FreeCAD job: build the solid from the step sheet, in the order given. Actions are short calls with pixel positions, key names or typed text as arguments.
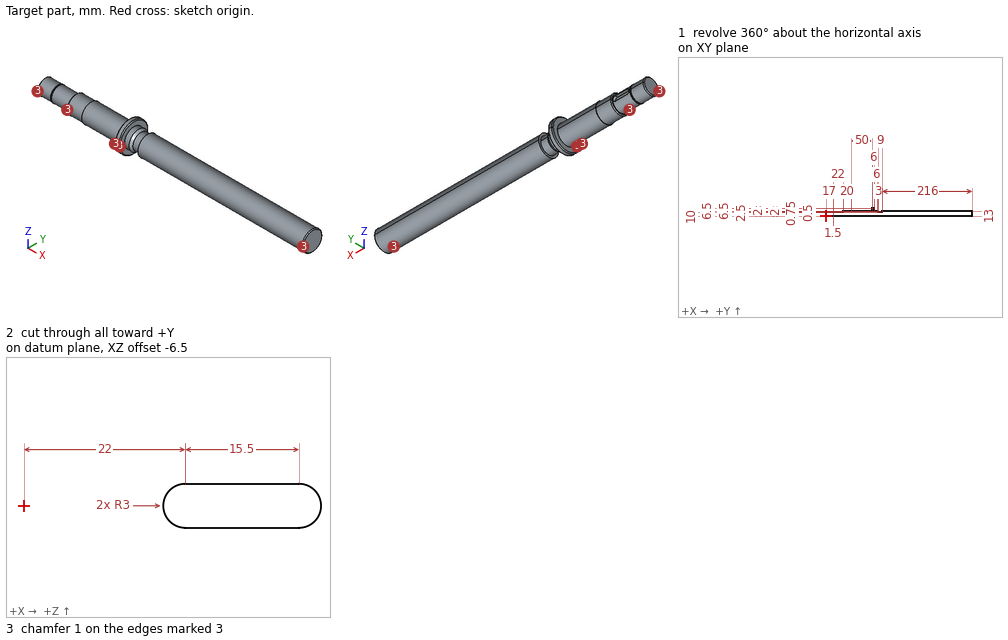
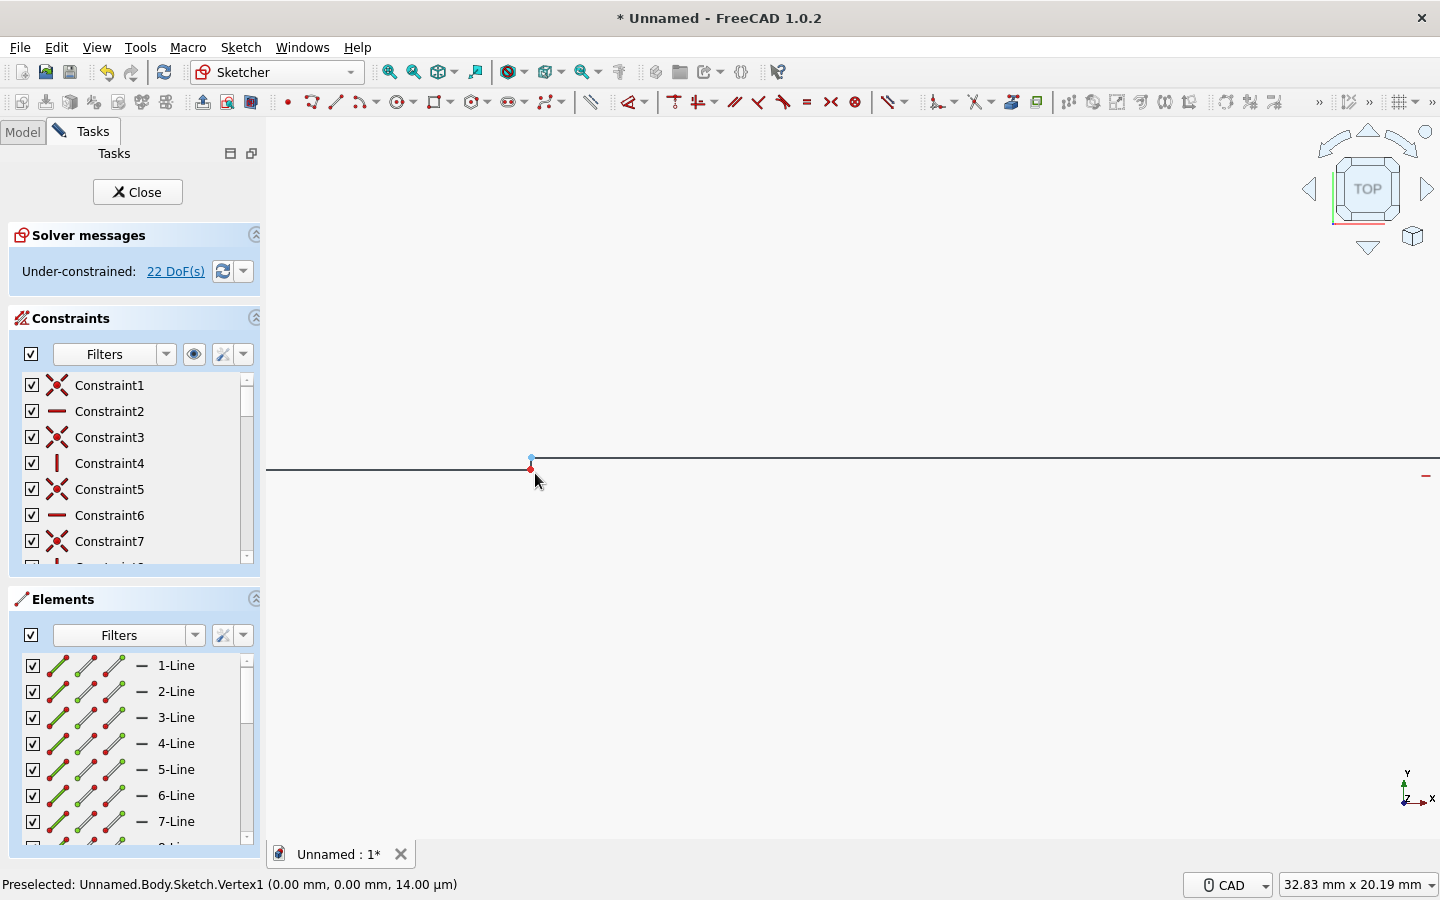
click(531, 464)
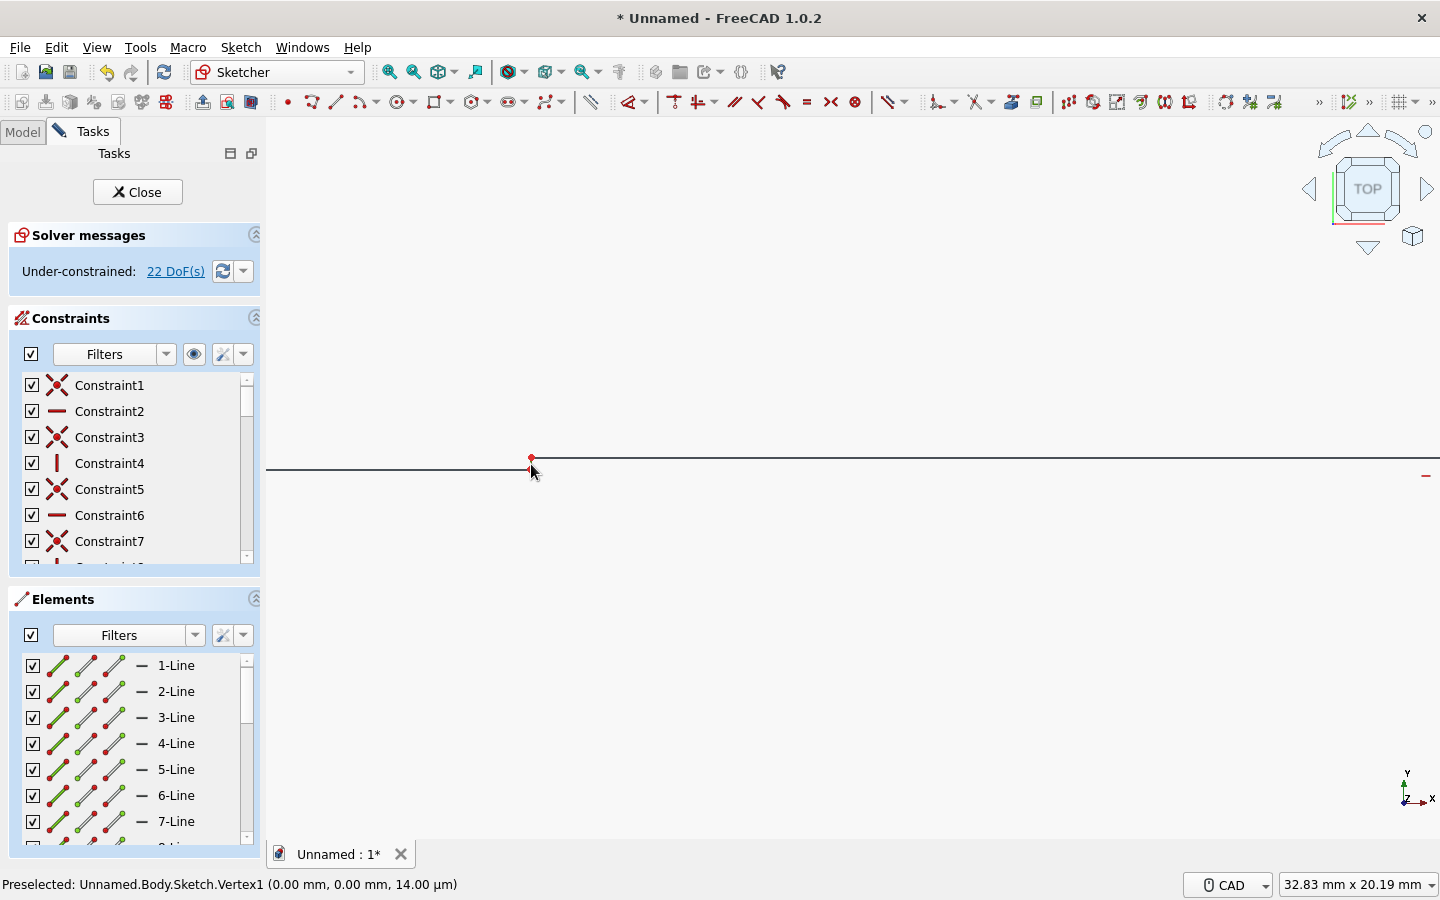
key(v)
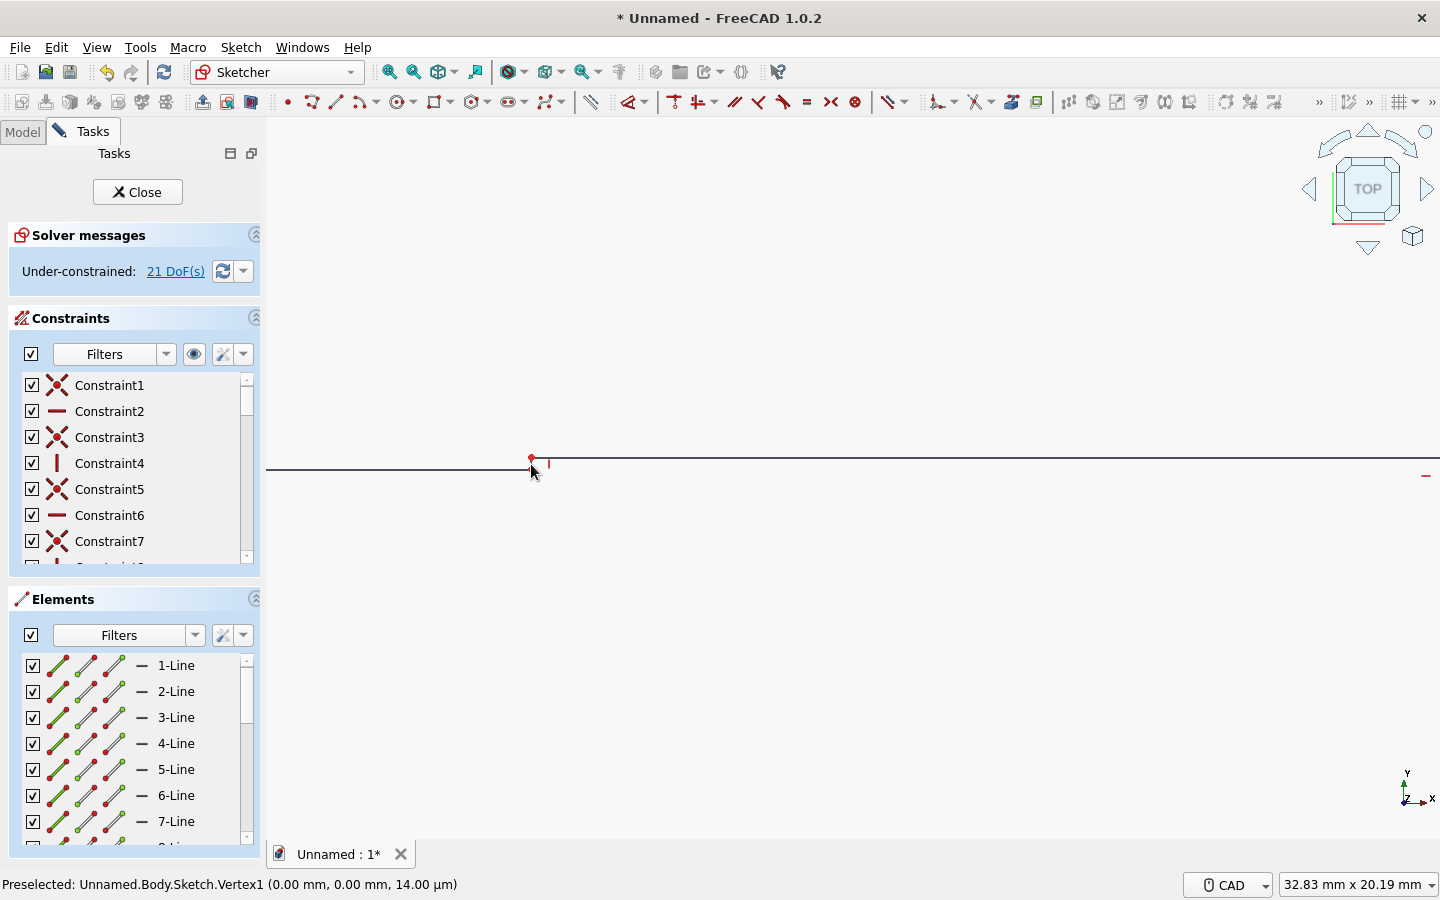
scroll(535, 473, down, 14)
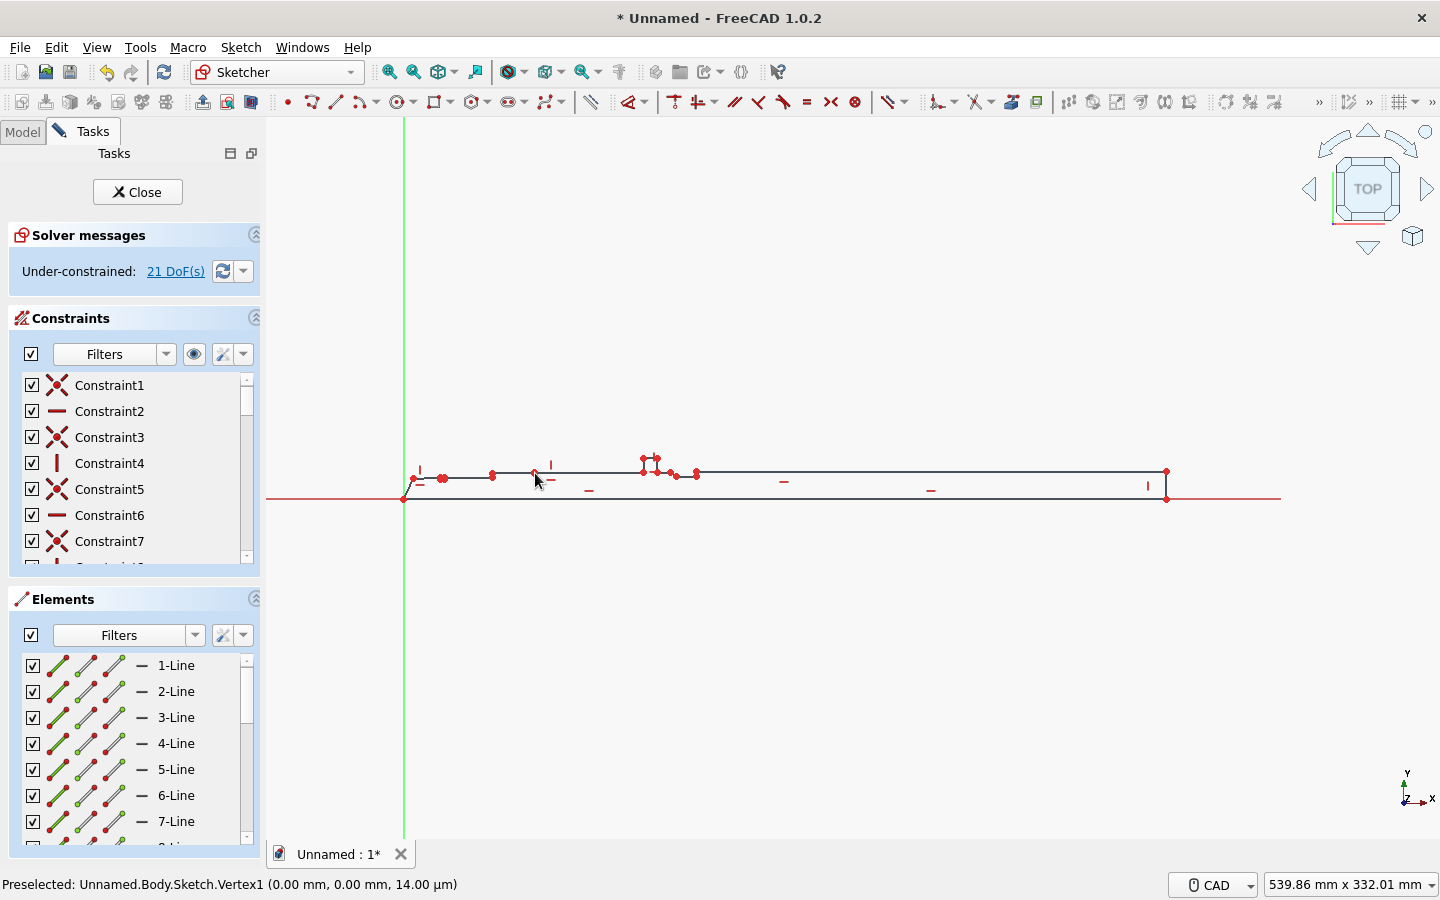
scroll(432, 478, up, 3)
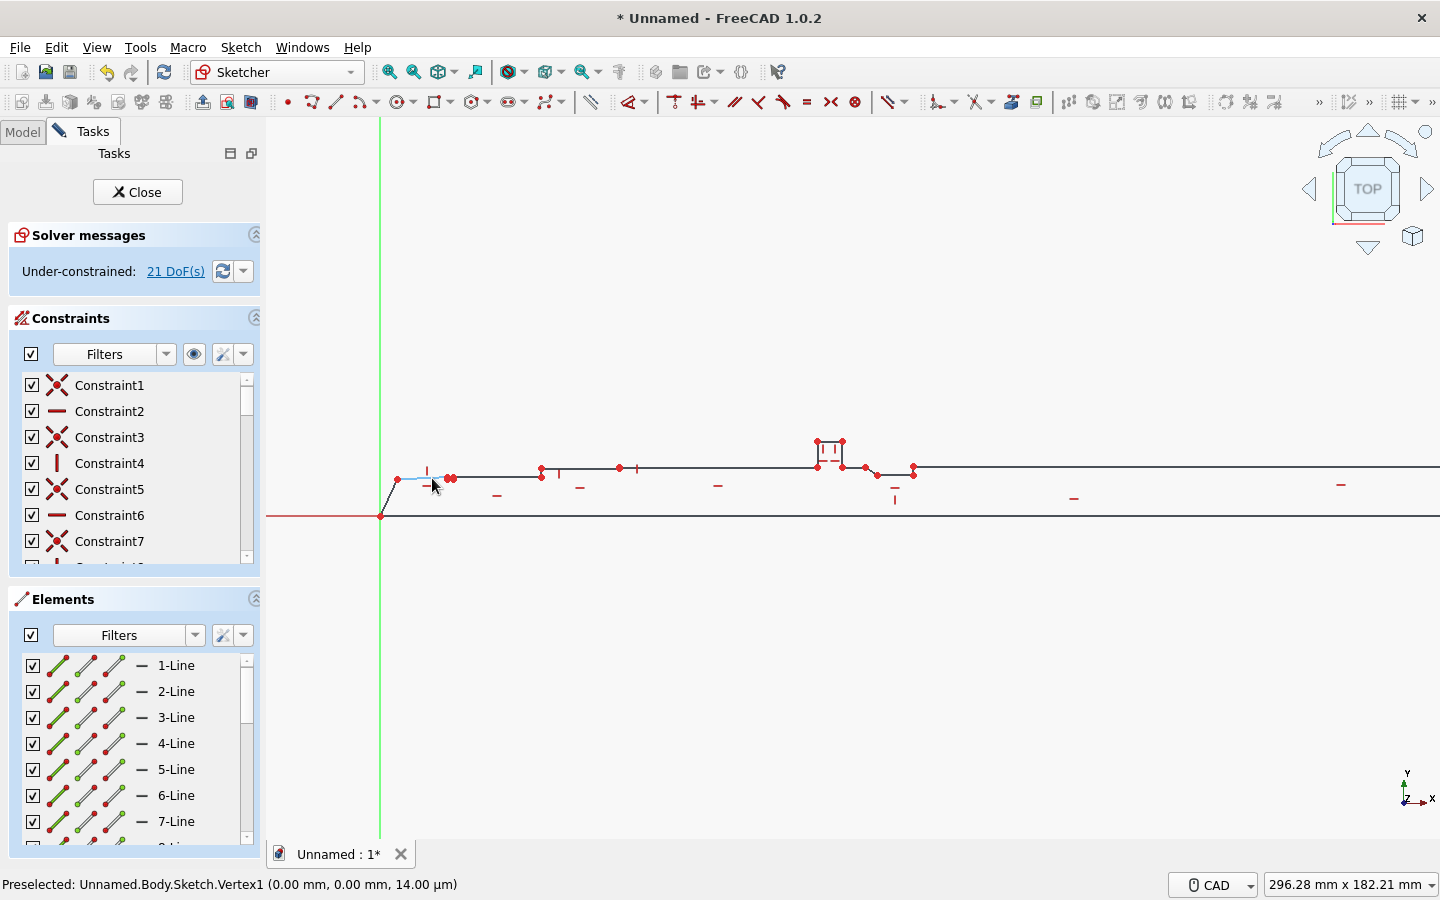
click(412, 479)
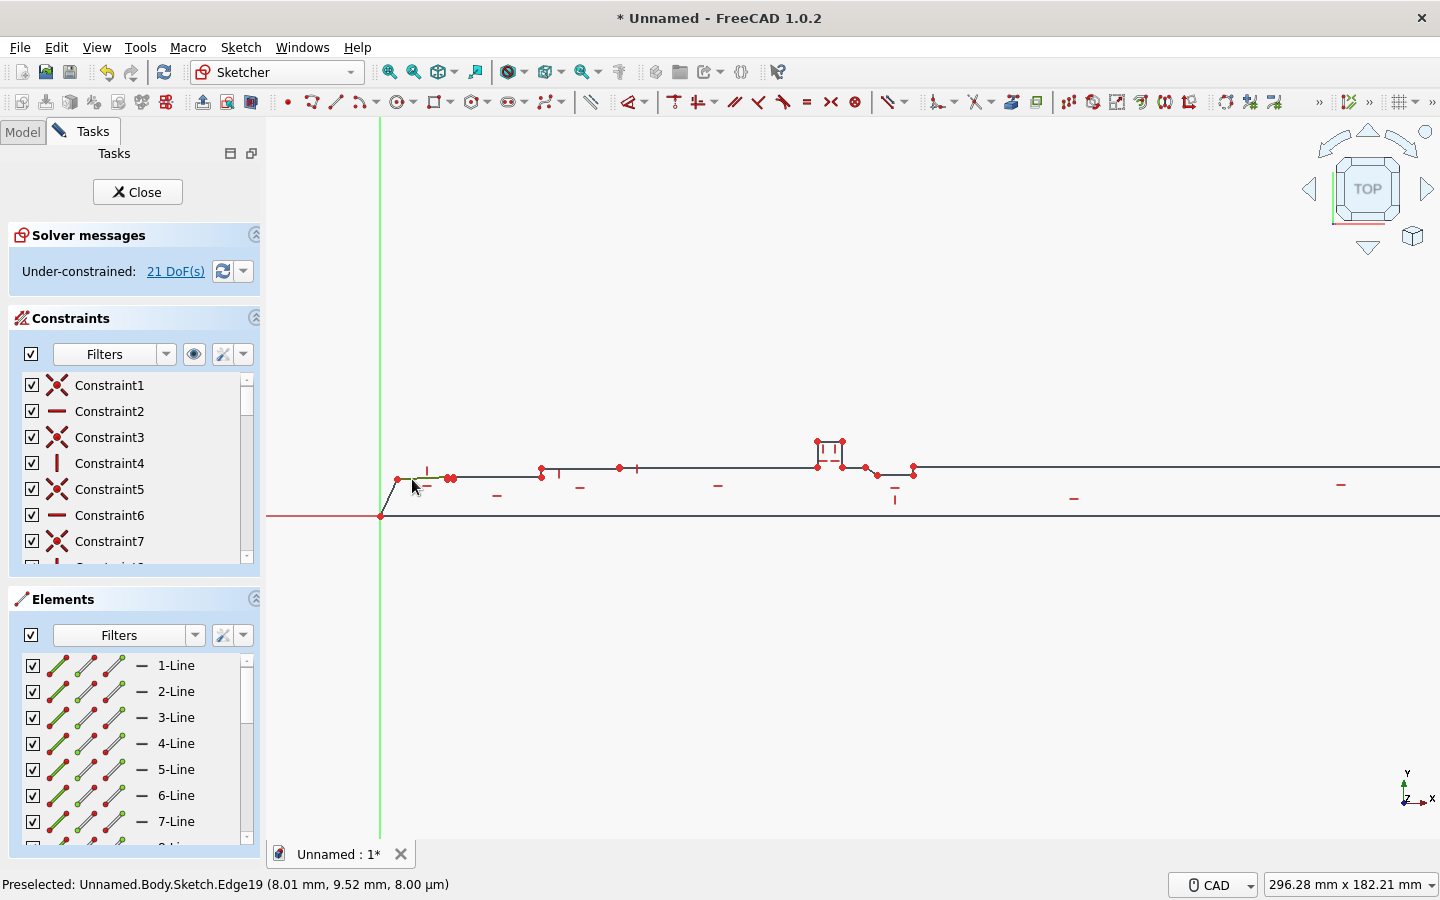
click(716, 102)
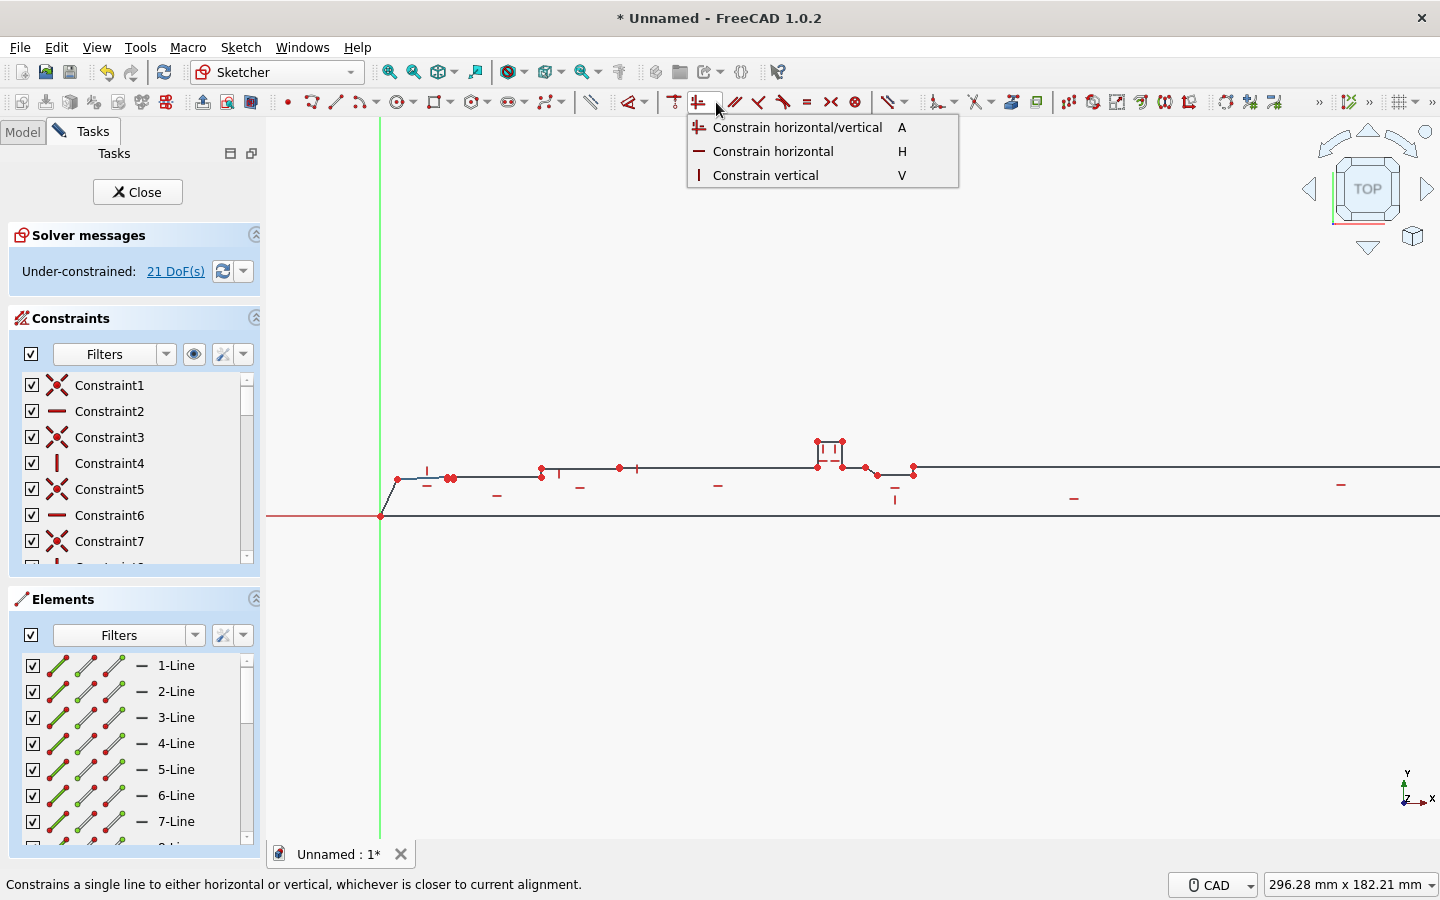
click(823, 151)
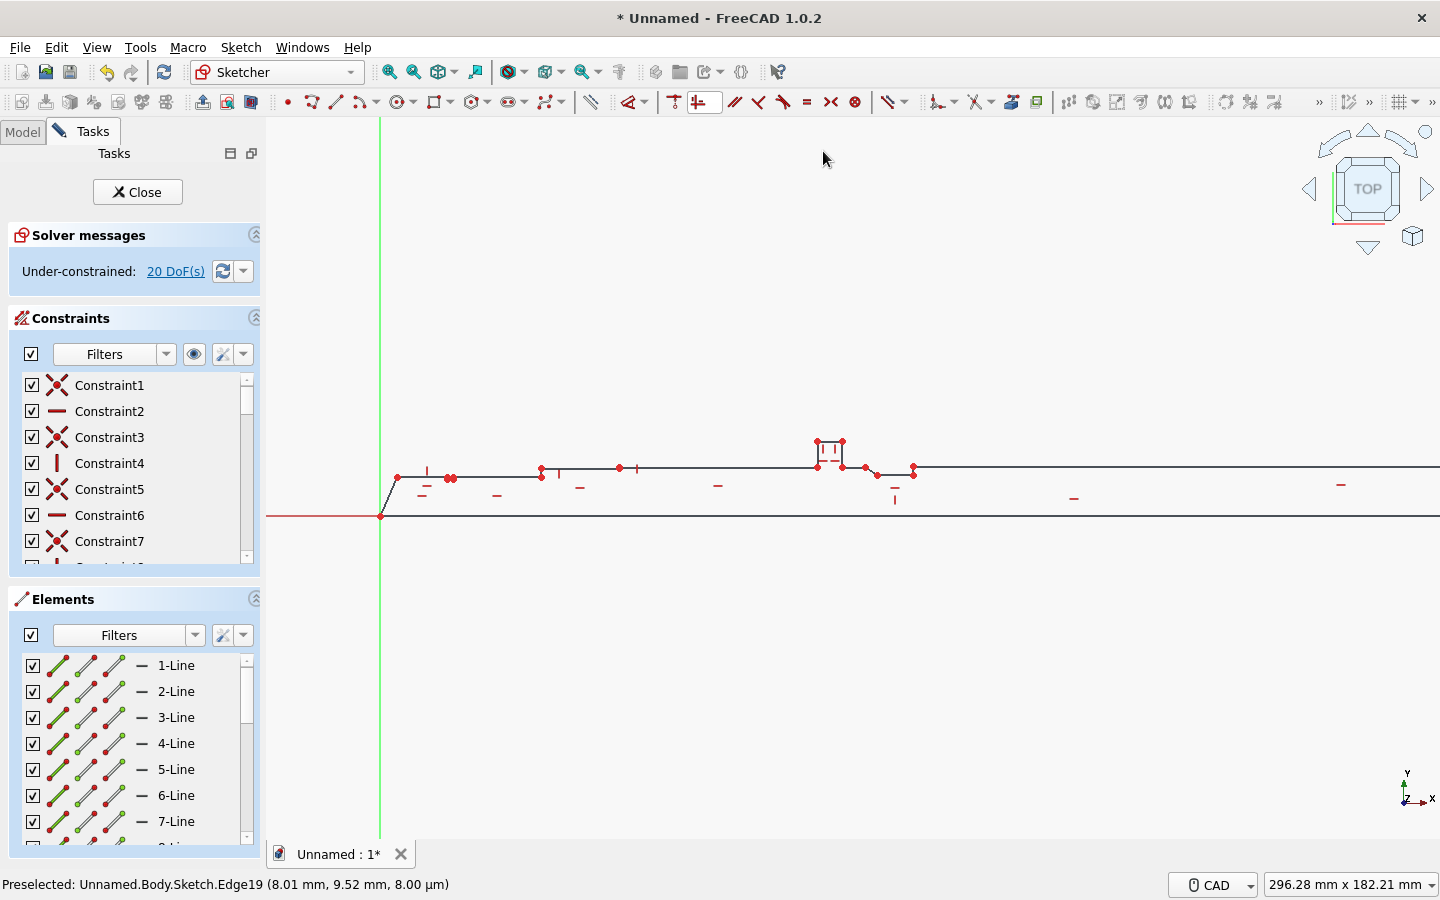
click(392, 489)